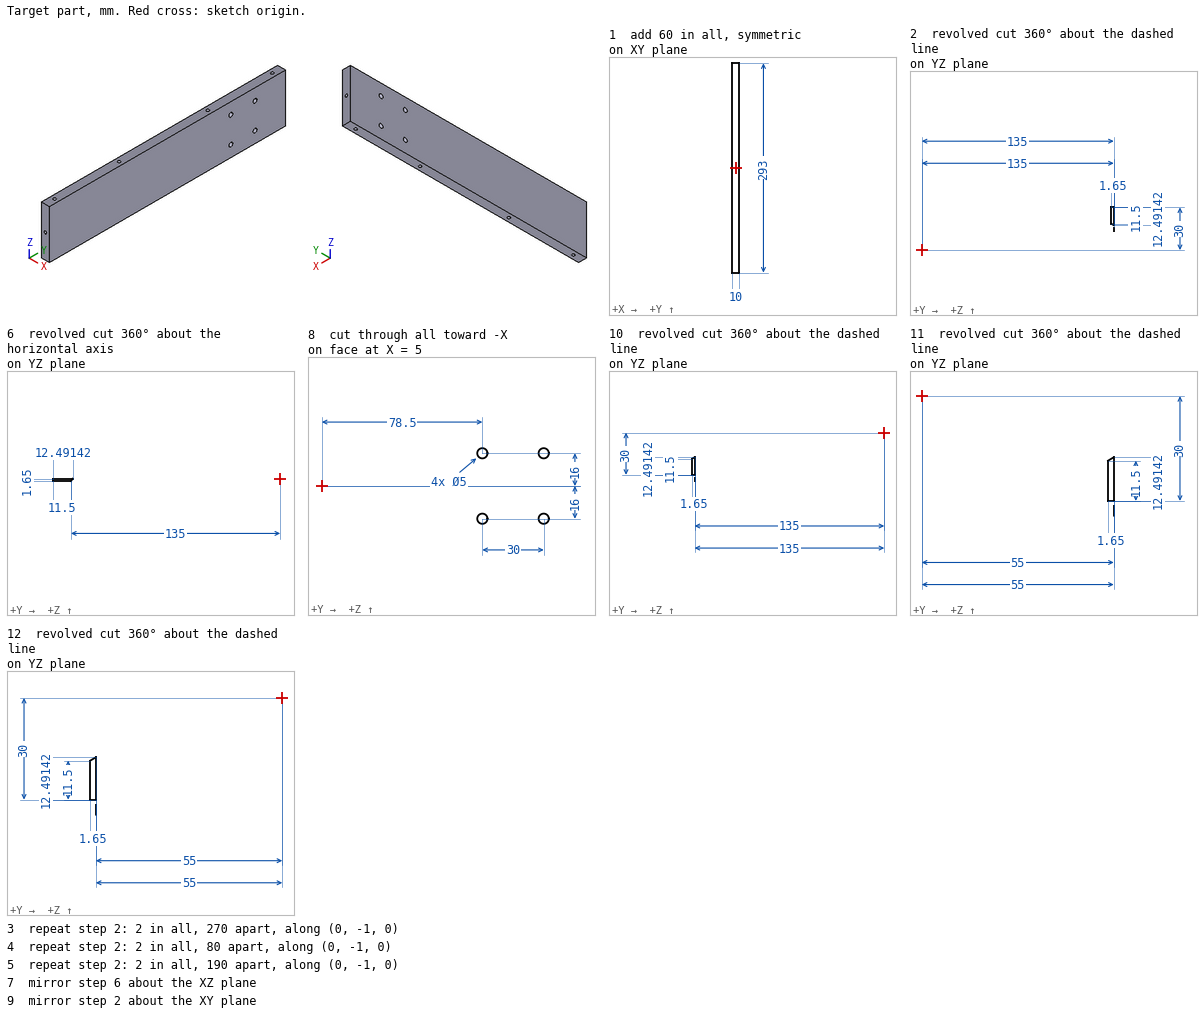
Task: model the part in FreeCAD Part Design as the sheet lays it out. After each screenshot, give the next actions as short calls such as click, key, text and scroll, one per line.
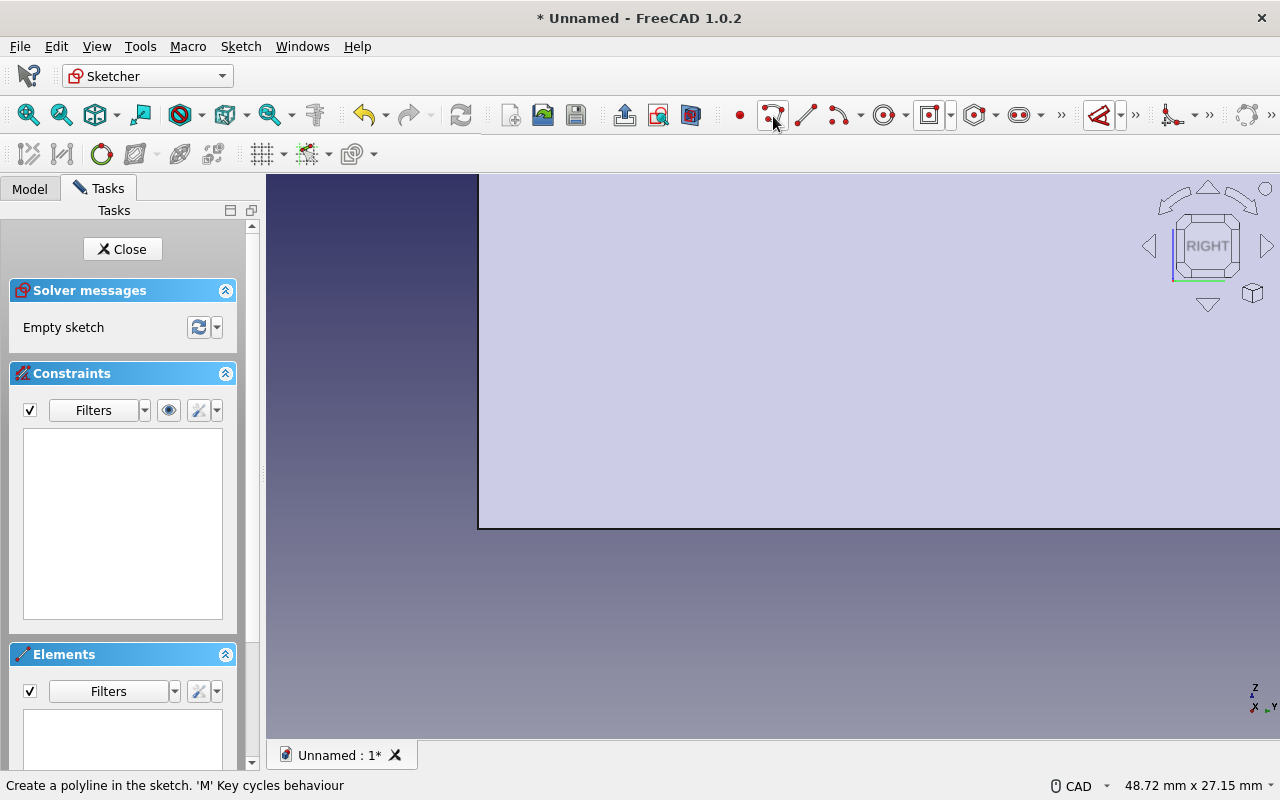
click(717, 269)
click(683, 289)
click(683, 529)
click(717, 529)
click(717, 270)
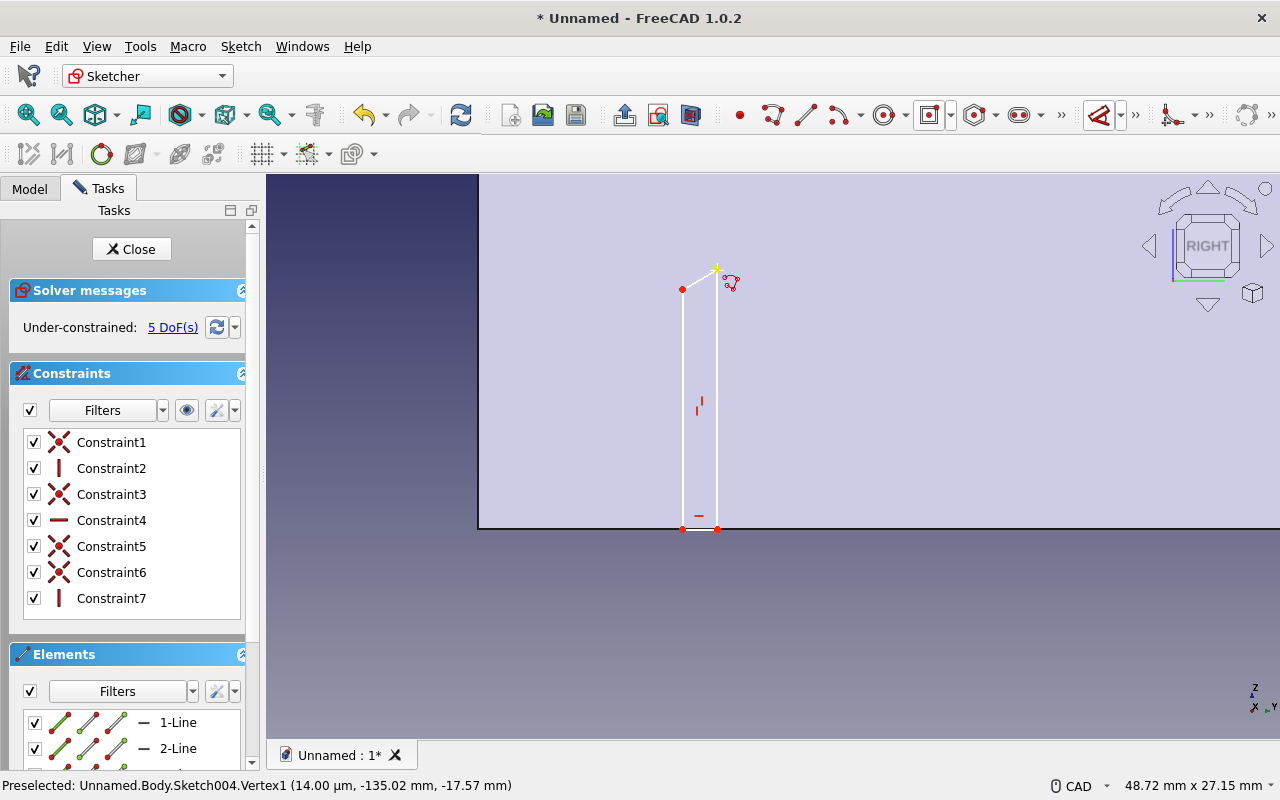
click(806, 116)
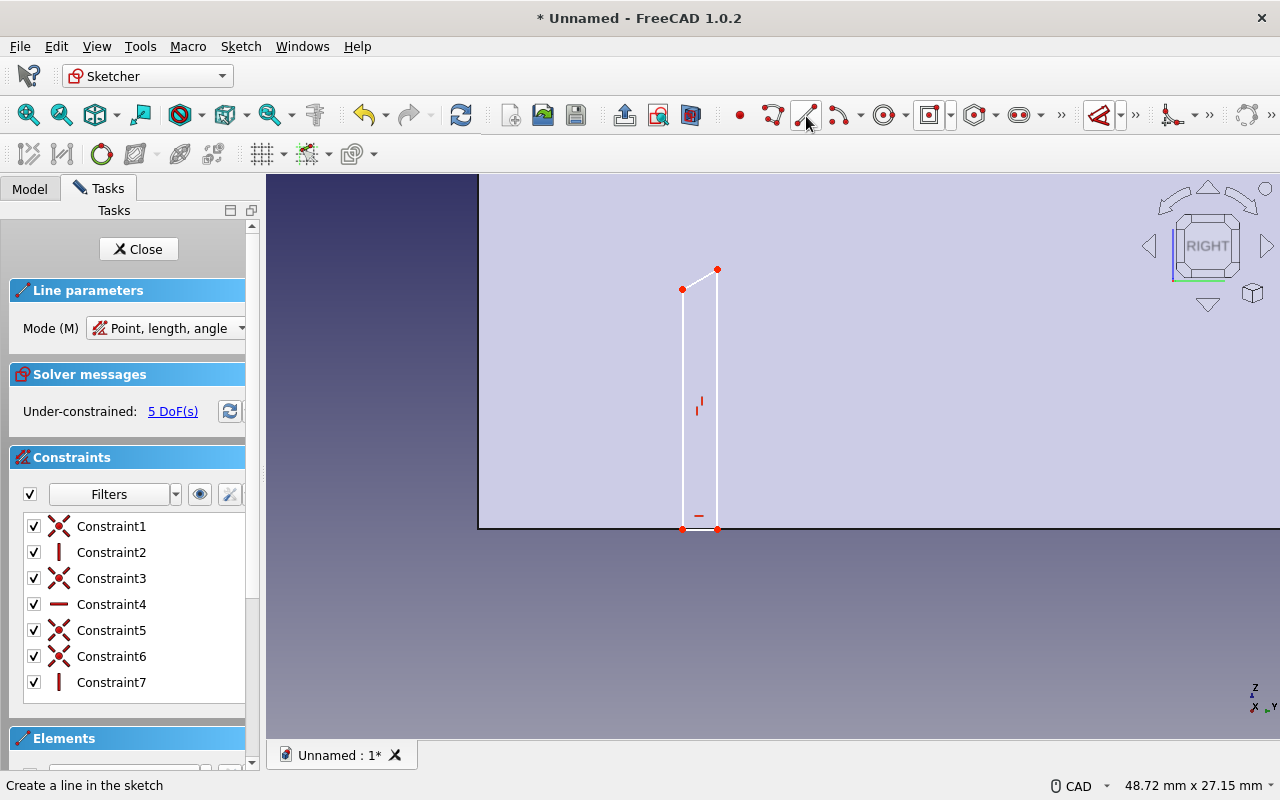
click(717, 555)
click(717, 633)
key(Escape)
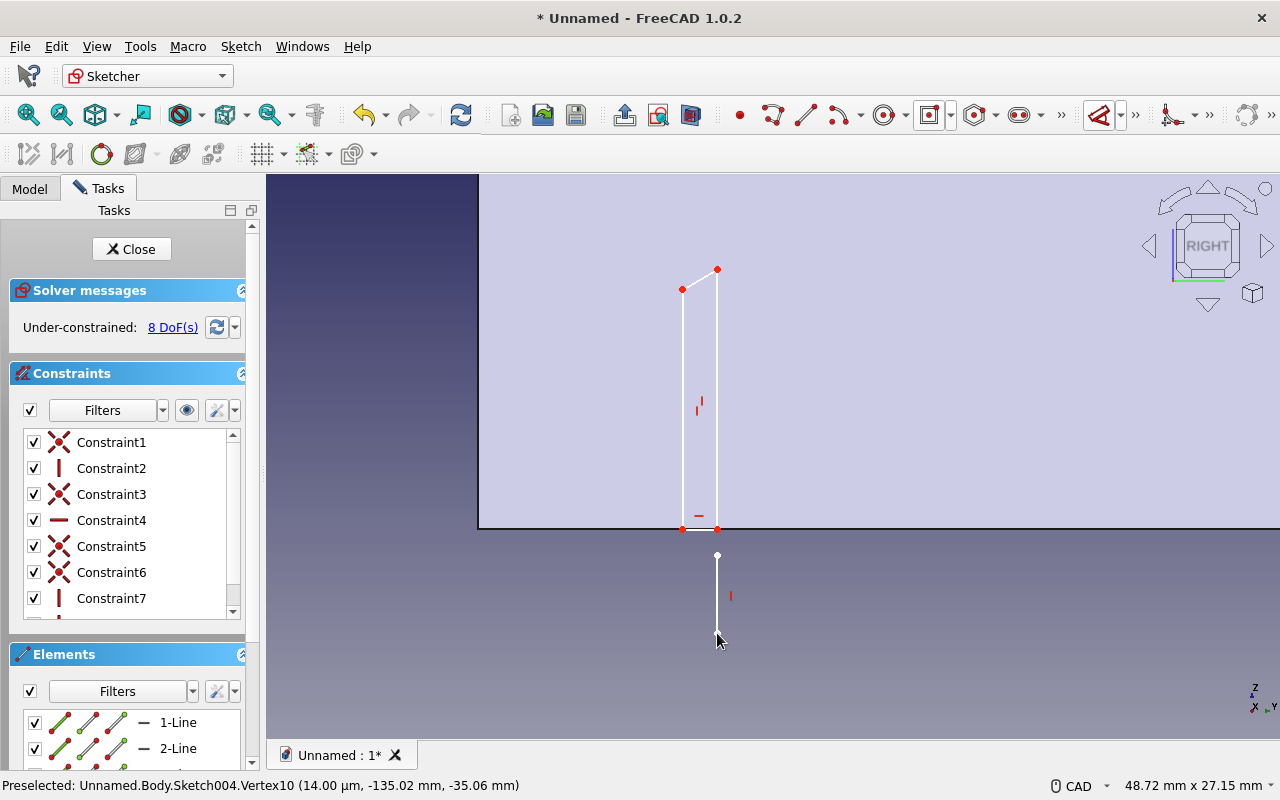
click(717, 579)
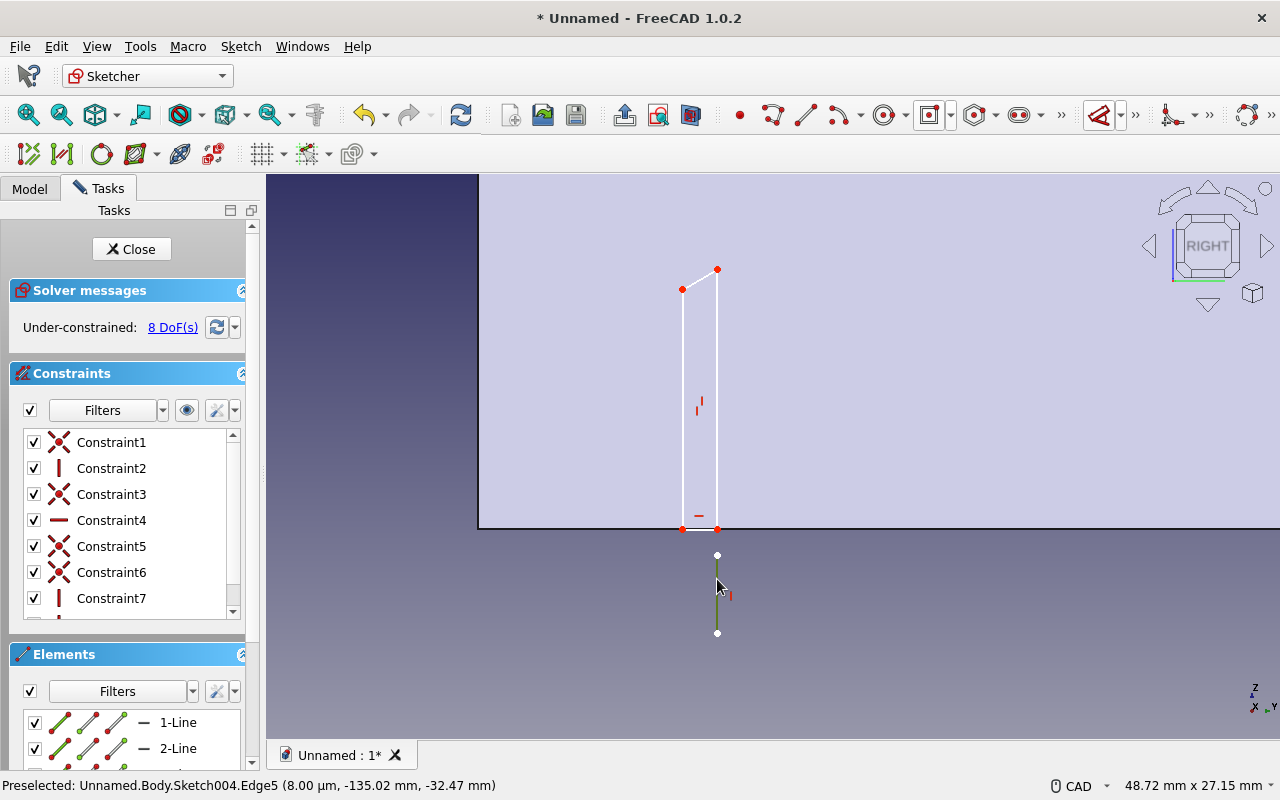
key(g)
key(n)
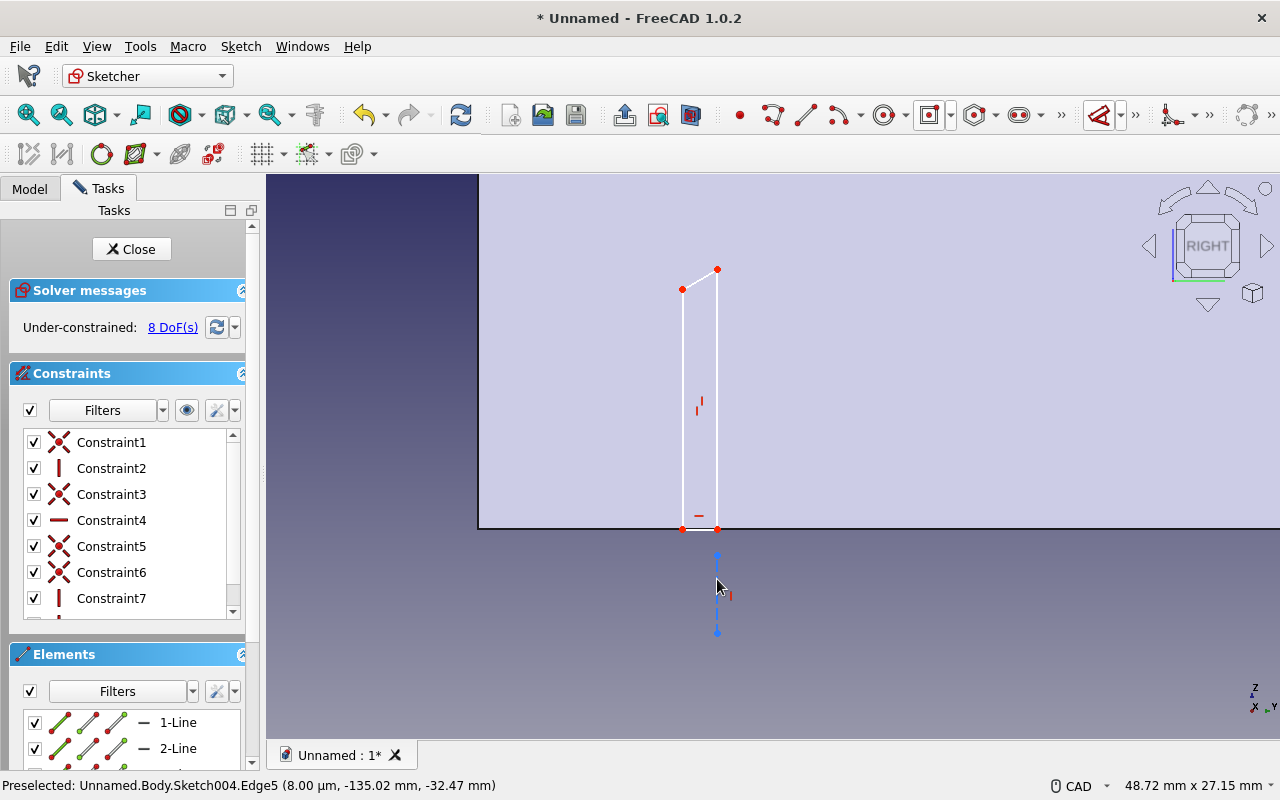
click(683, 530)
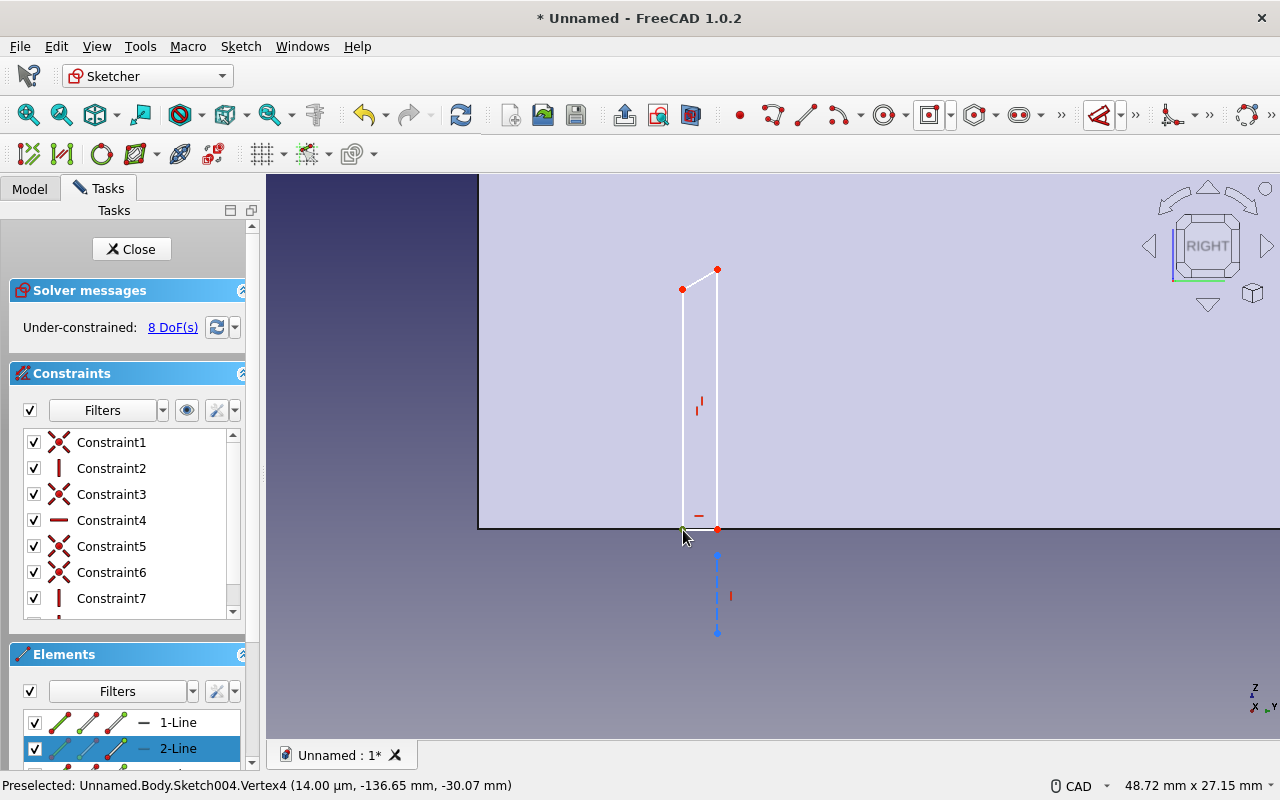
click(1120, 116)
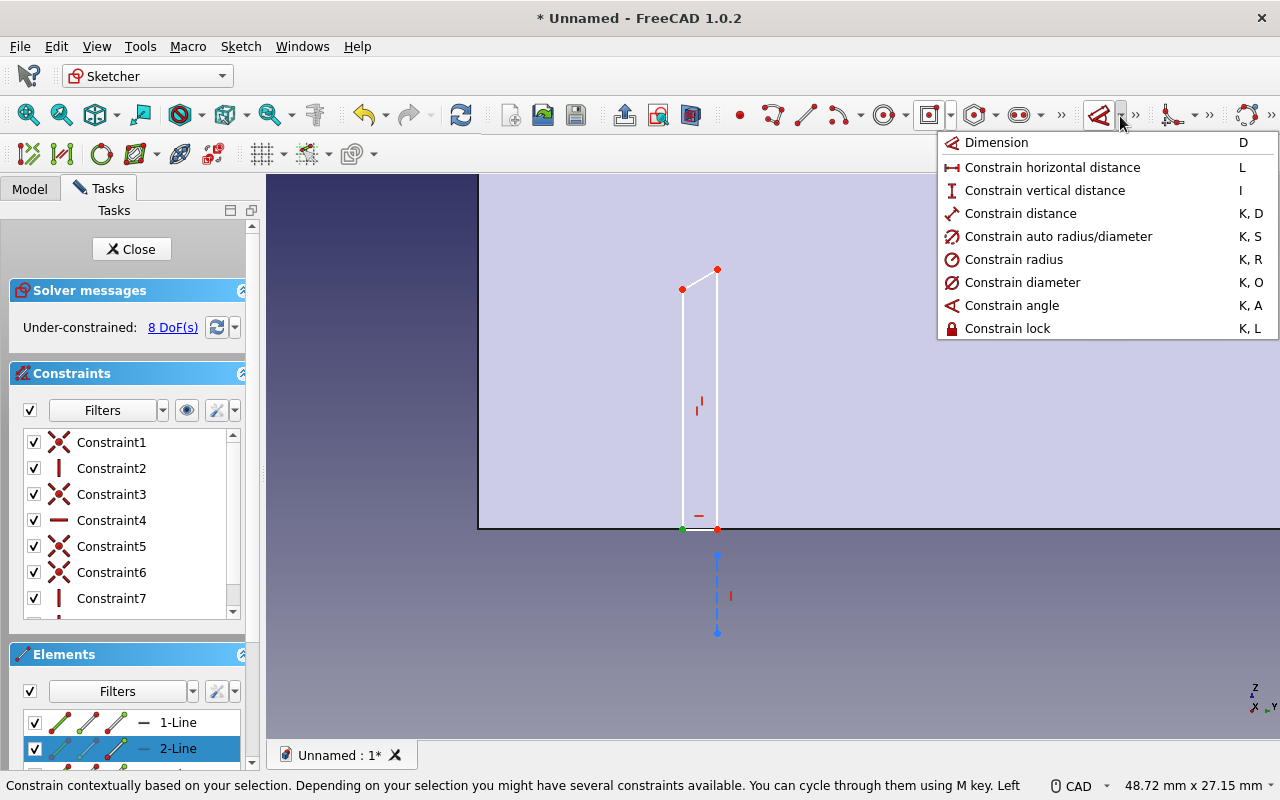
click(1108, 190)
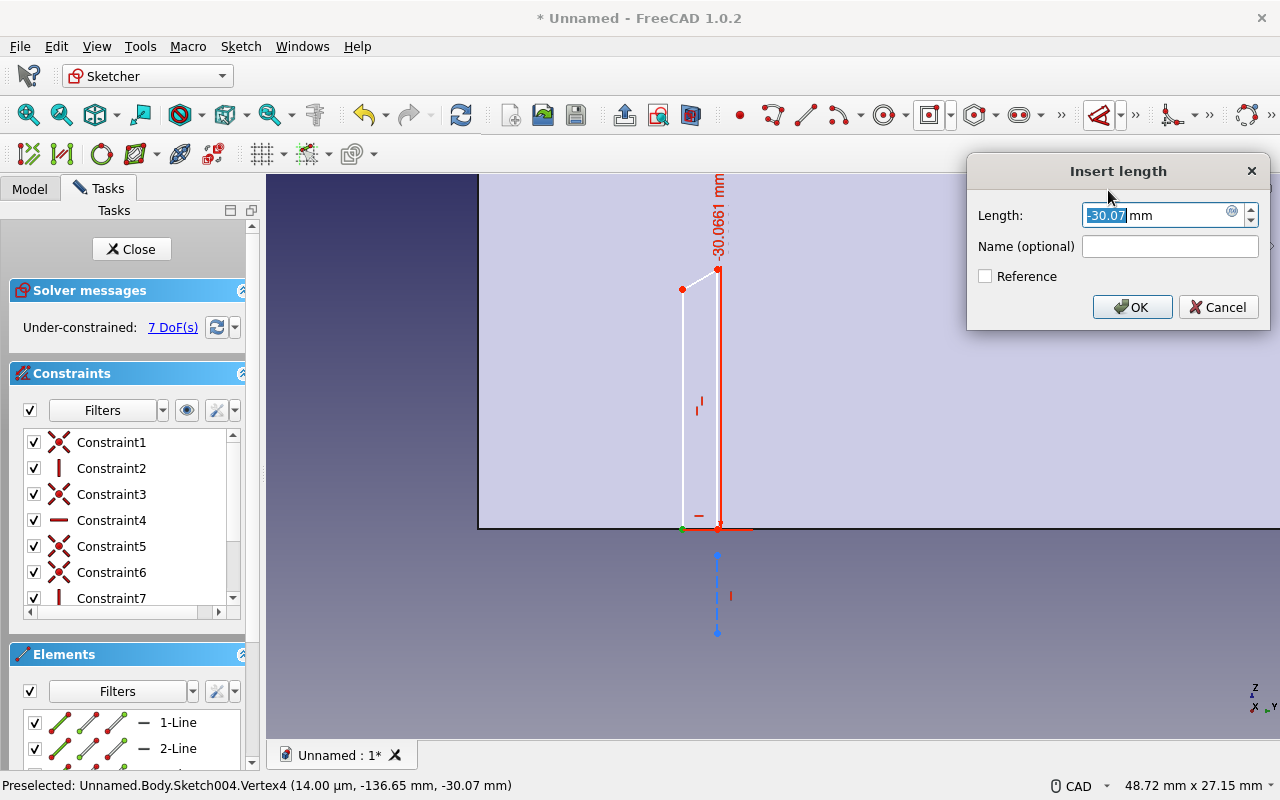
text(-30)
key(Return)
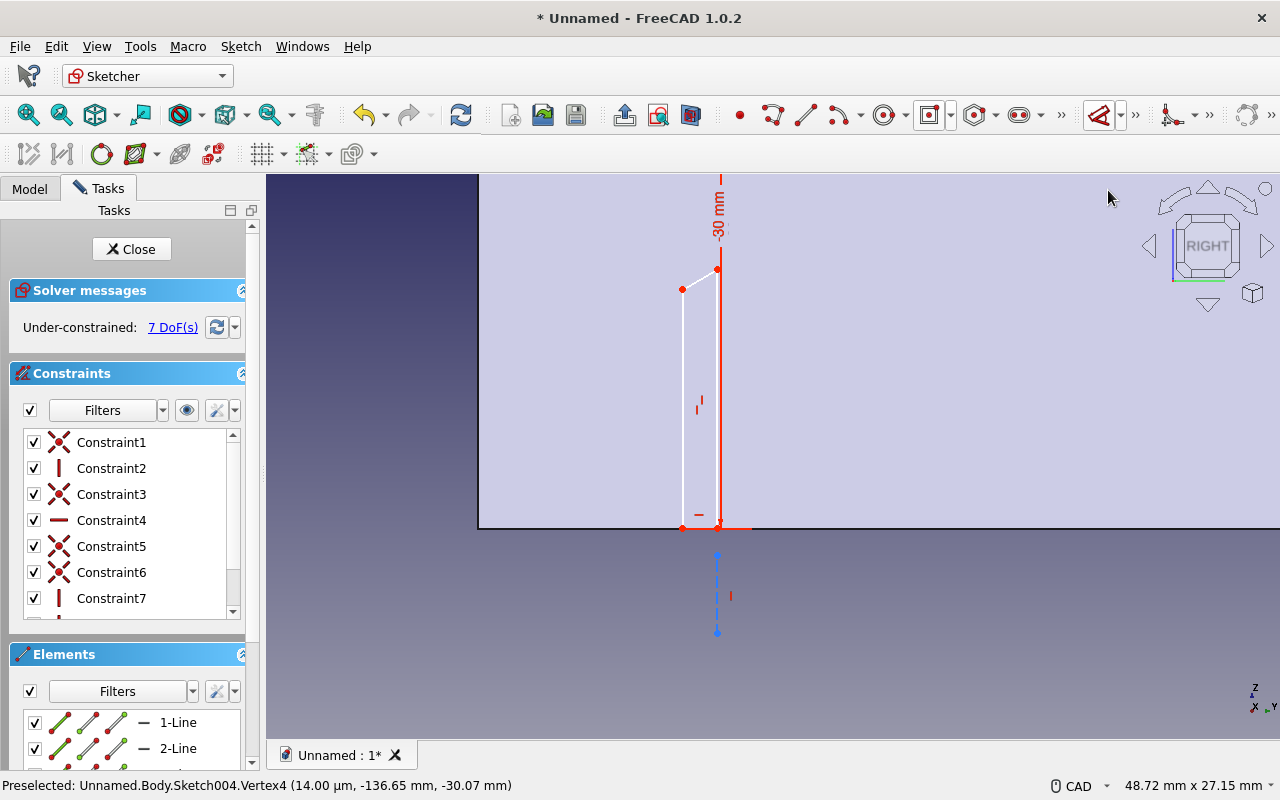
click(683, 362)